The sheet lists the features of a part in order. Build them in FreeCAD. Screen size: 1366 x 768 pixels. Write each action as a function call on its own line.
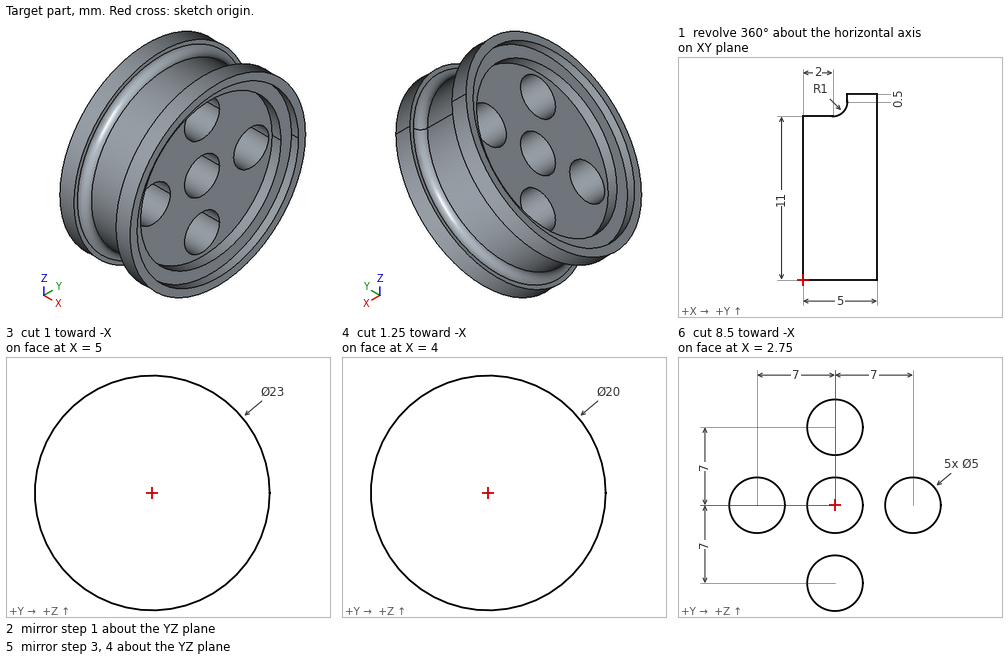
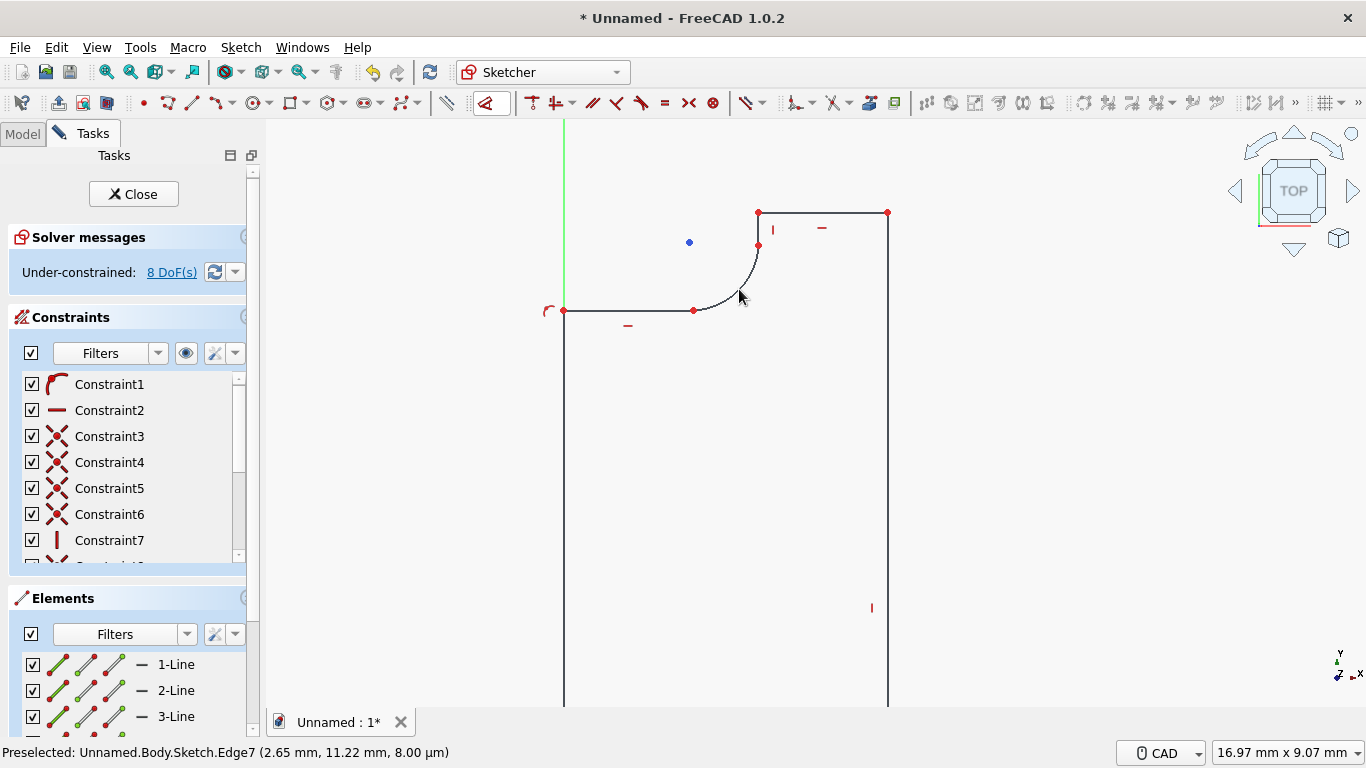
click(655, 311)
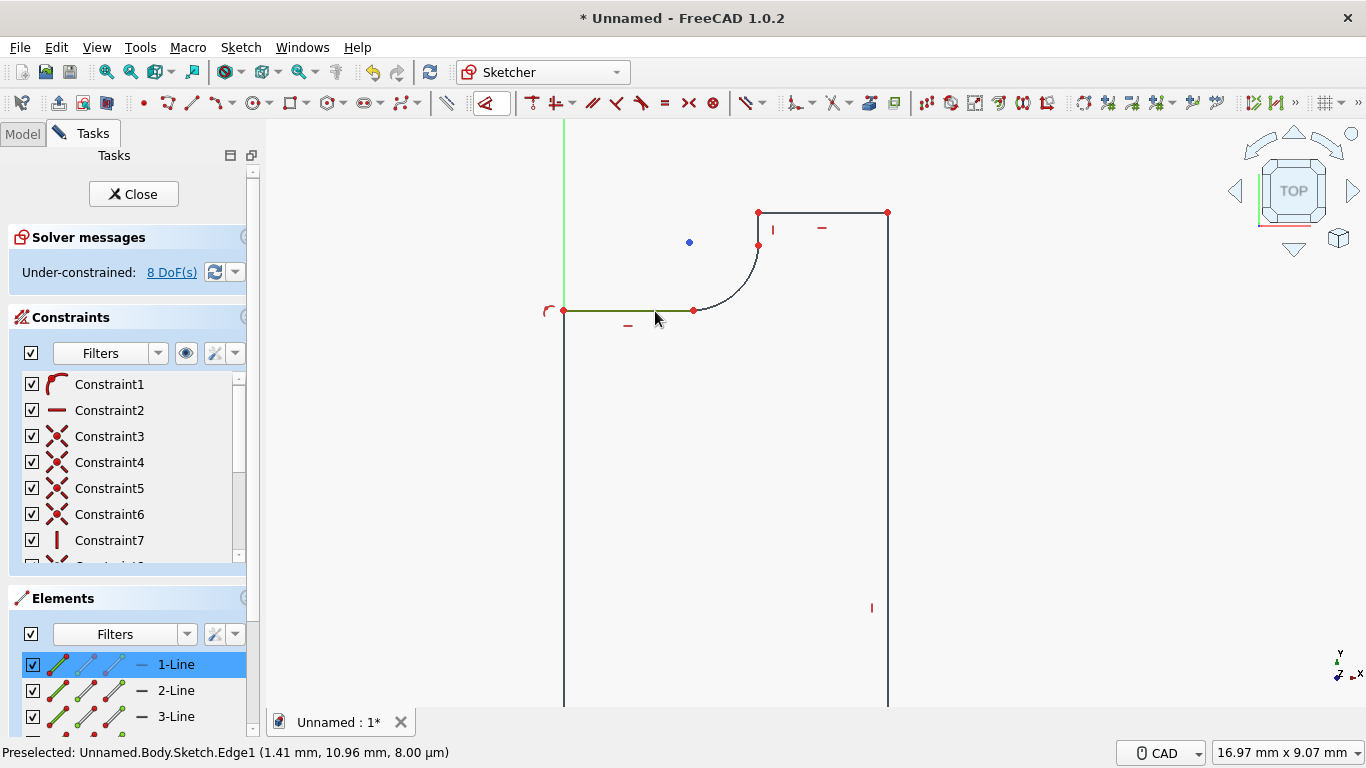
click(723, 302)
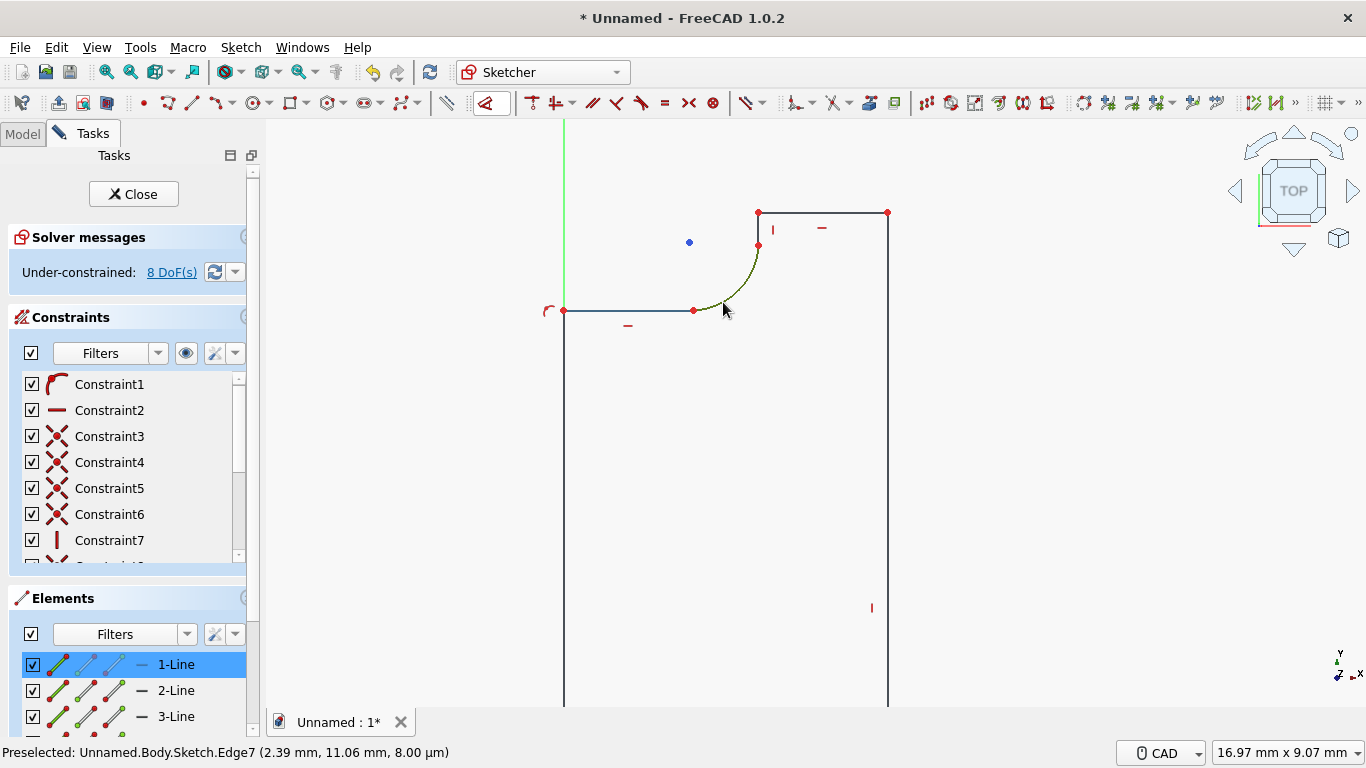
key(t)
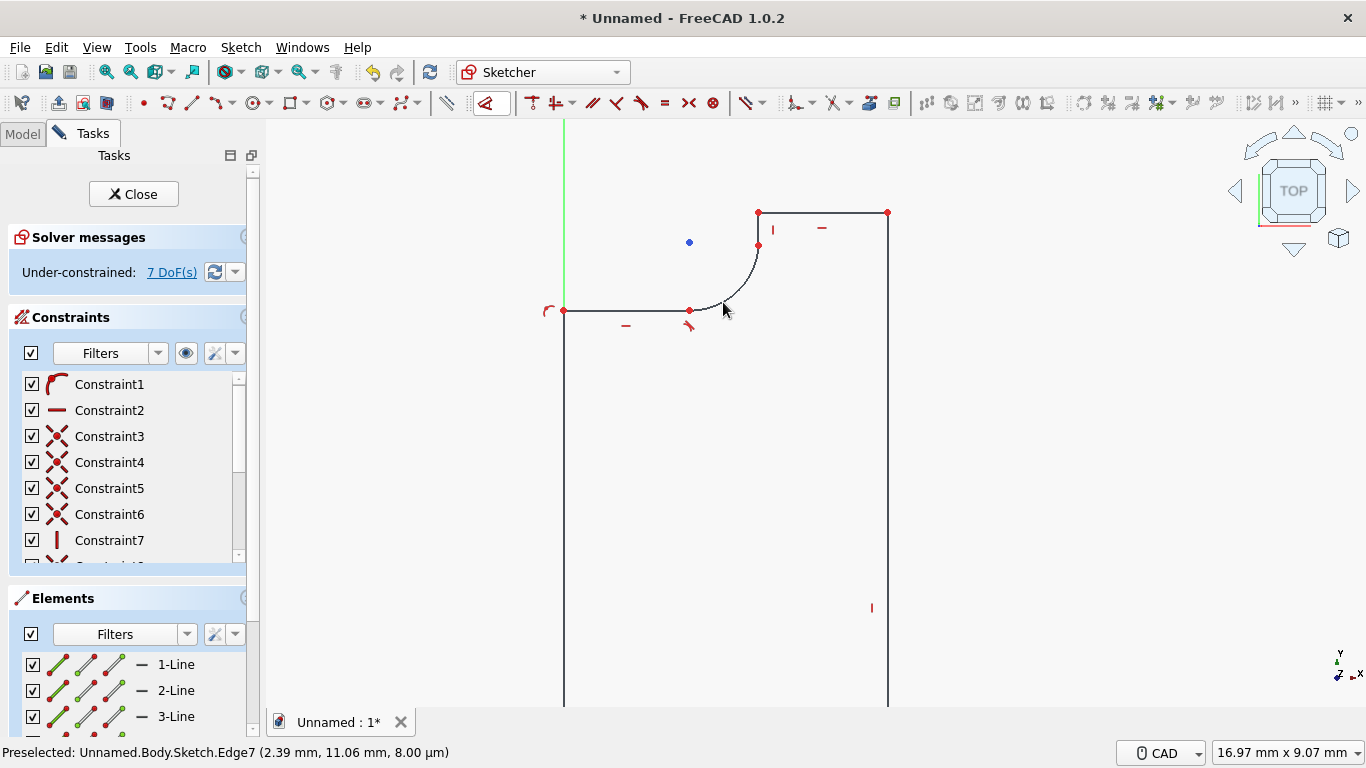
scroll(758, 223, up, 2)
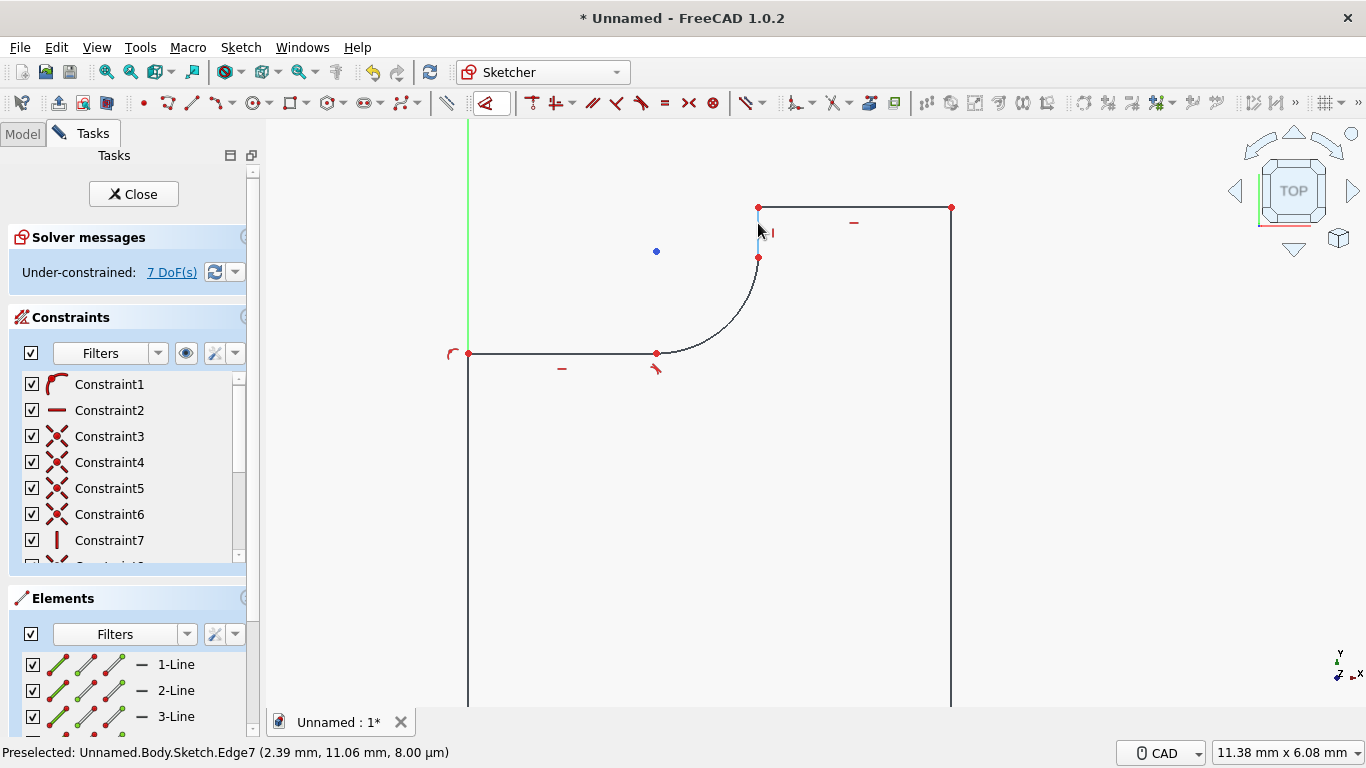
click(758, 222)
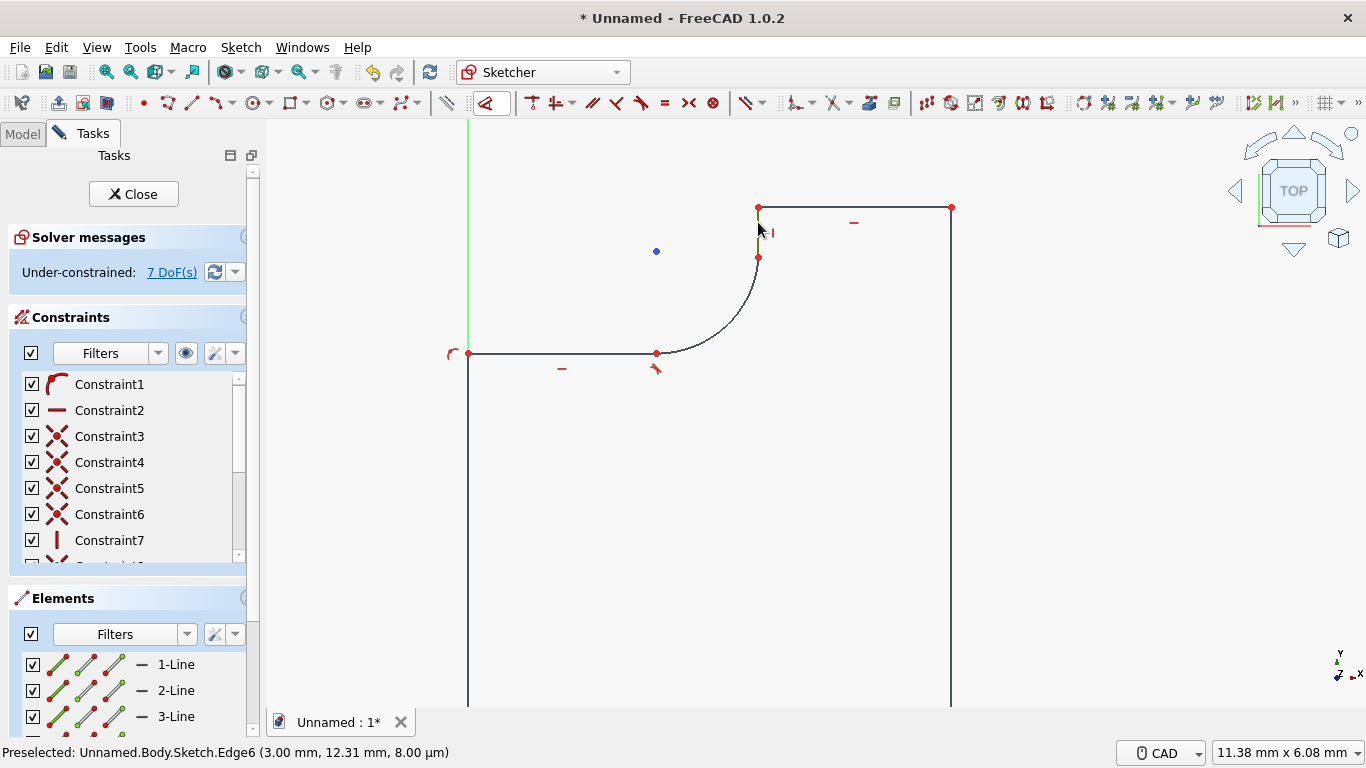
click(701, 343)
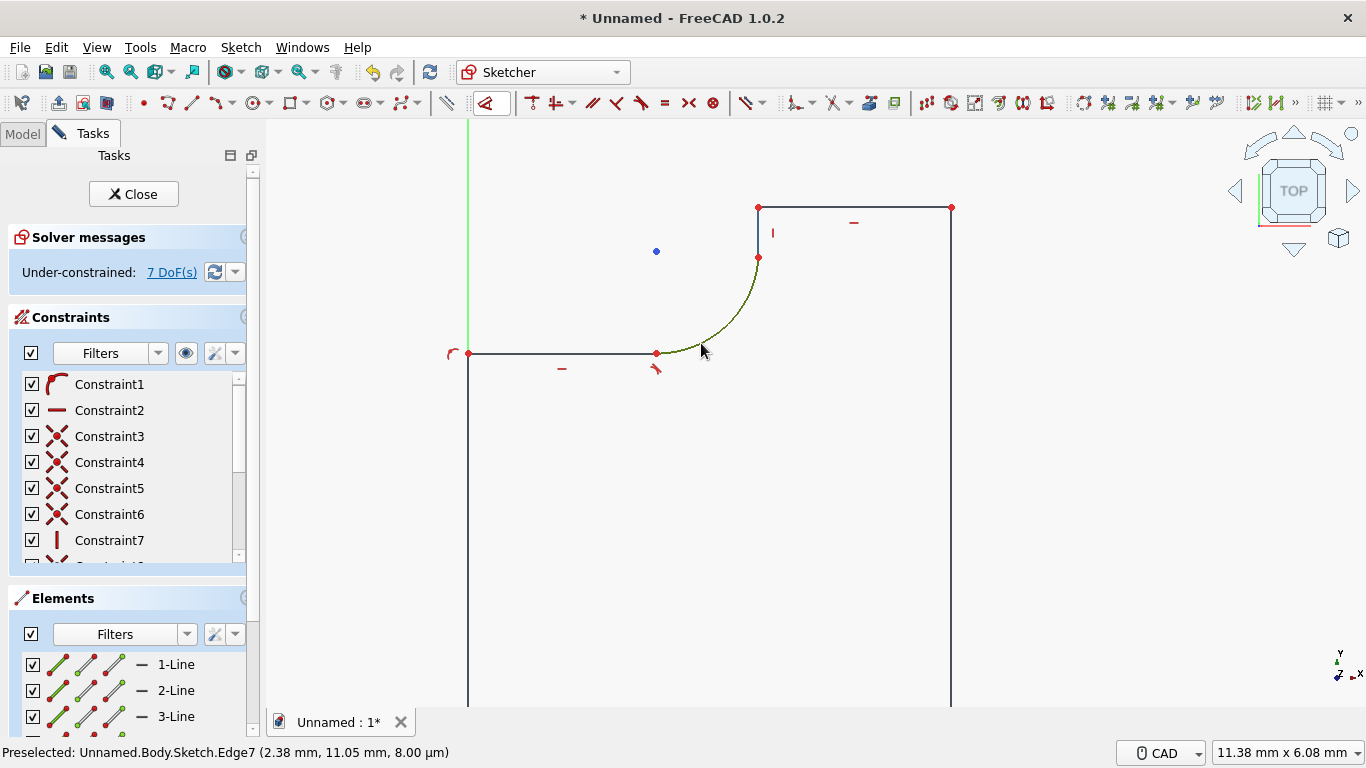
key(t)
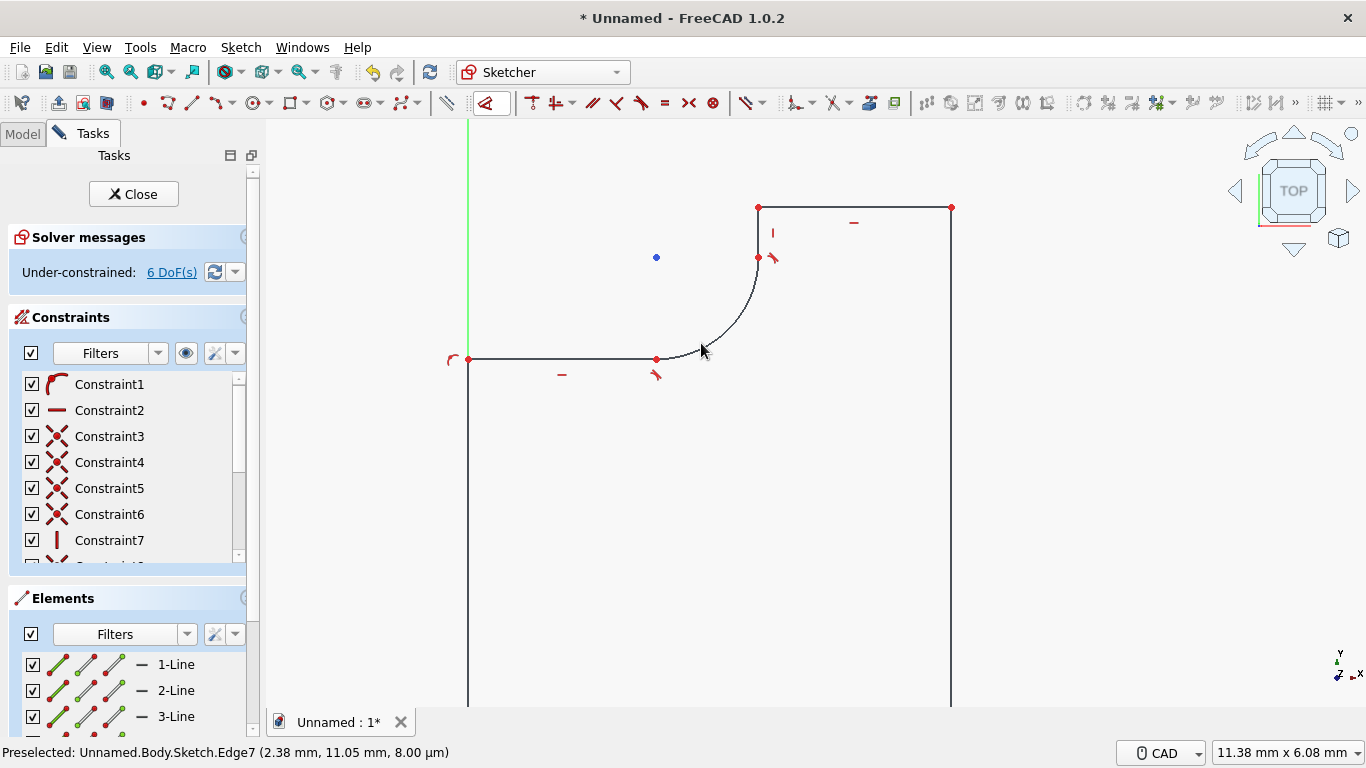
scroll(764, 242, down, 6)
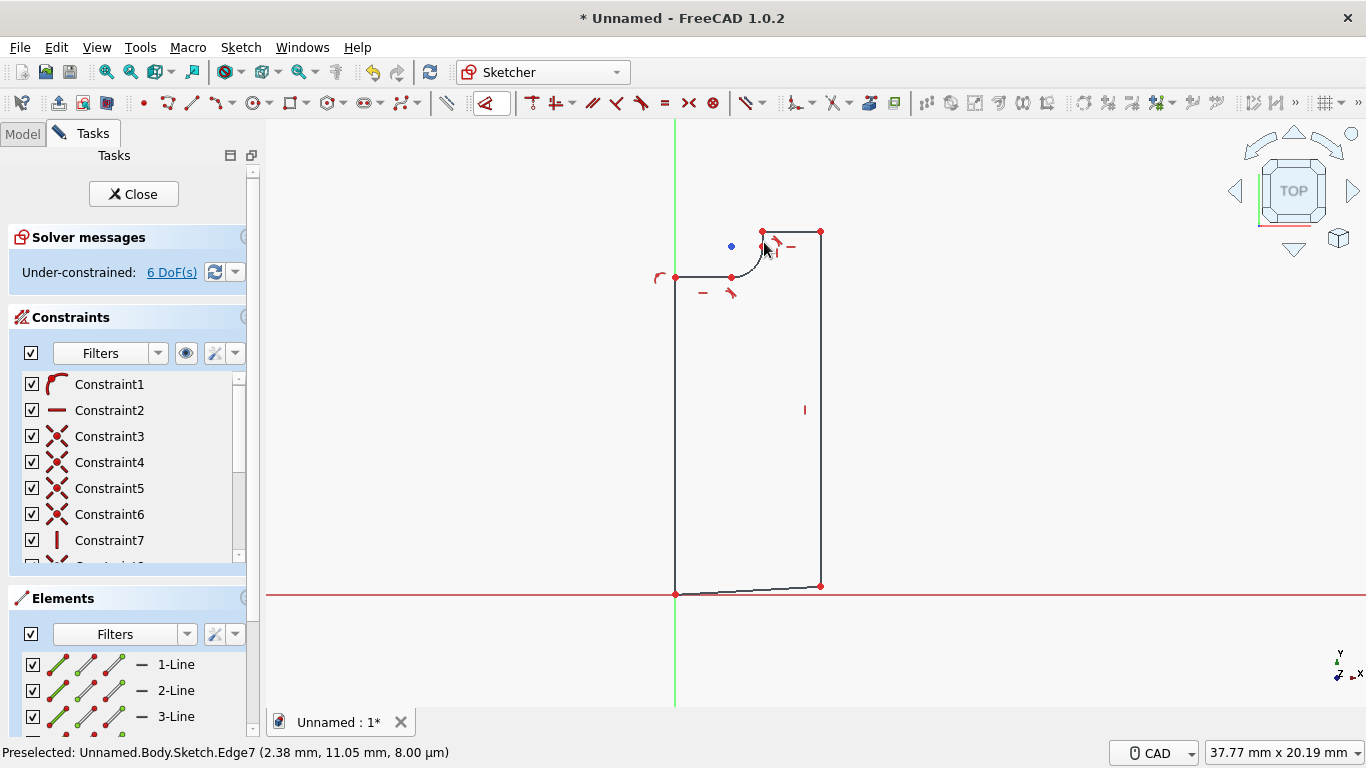
scroll(777, 589, up, 5)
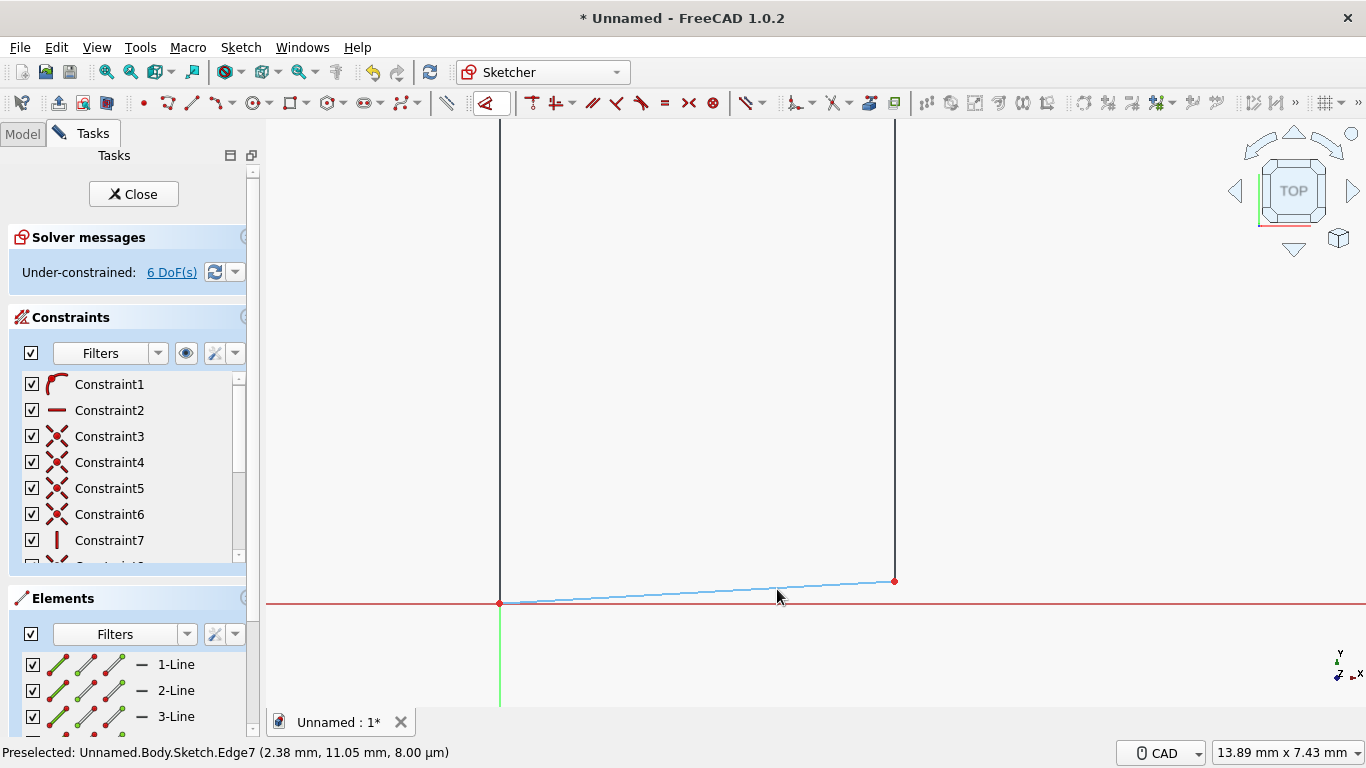
click(776, 588)